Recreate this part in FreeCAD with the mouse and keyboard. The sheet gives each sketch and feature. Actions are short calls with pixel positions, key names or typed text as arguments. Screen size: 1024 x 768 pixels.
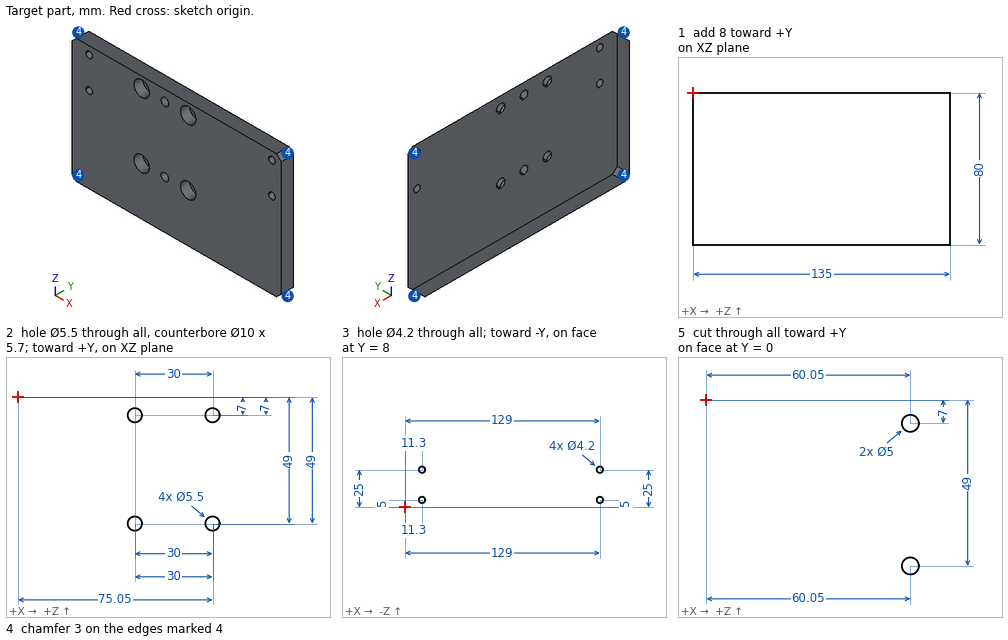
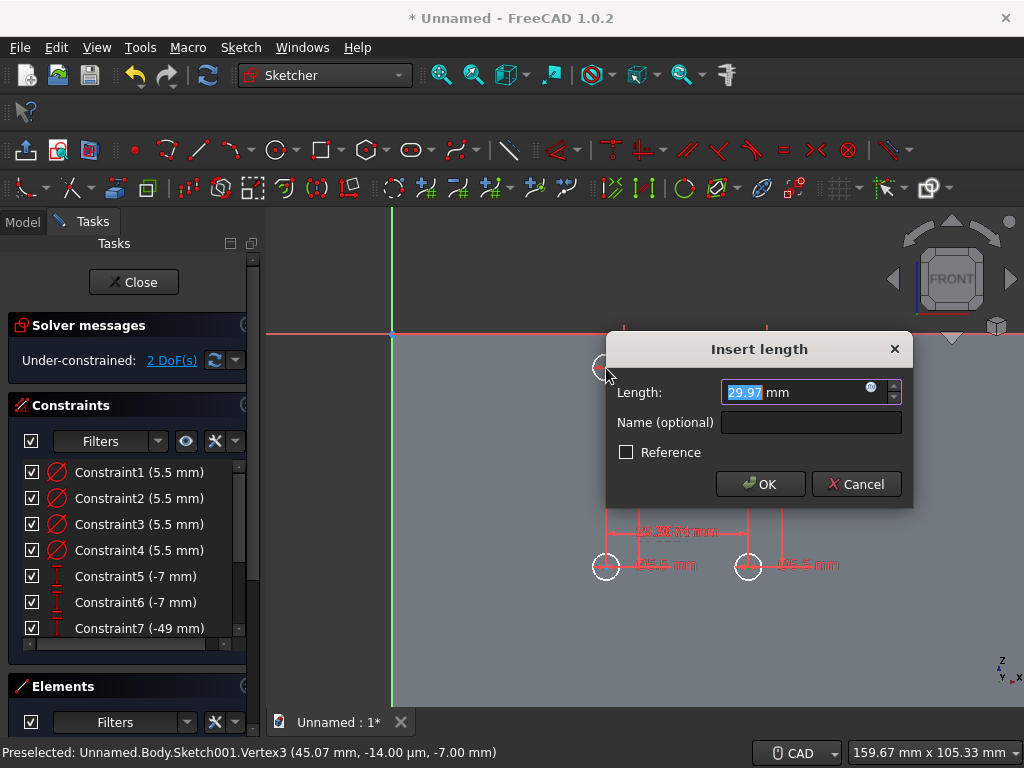
text(30)
key(Return)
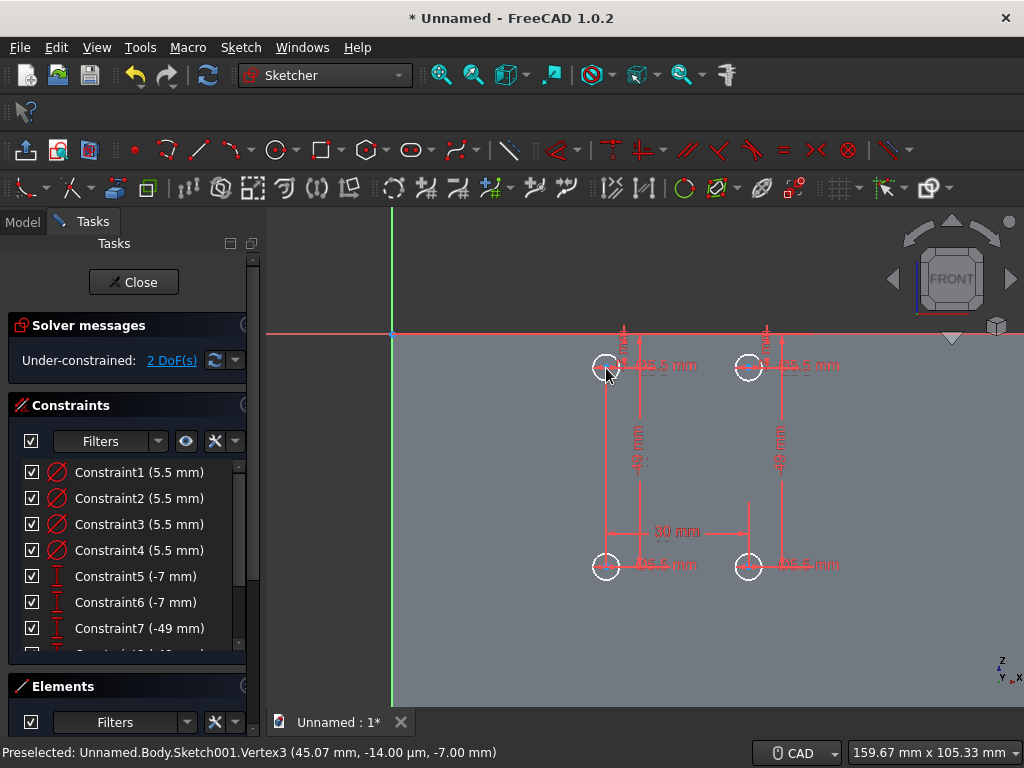
click(606, 368)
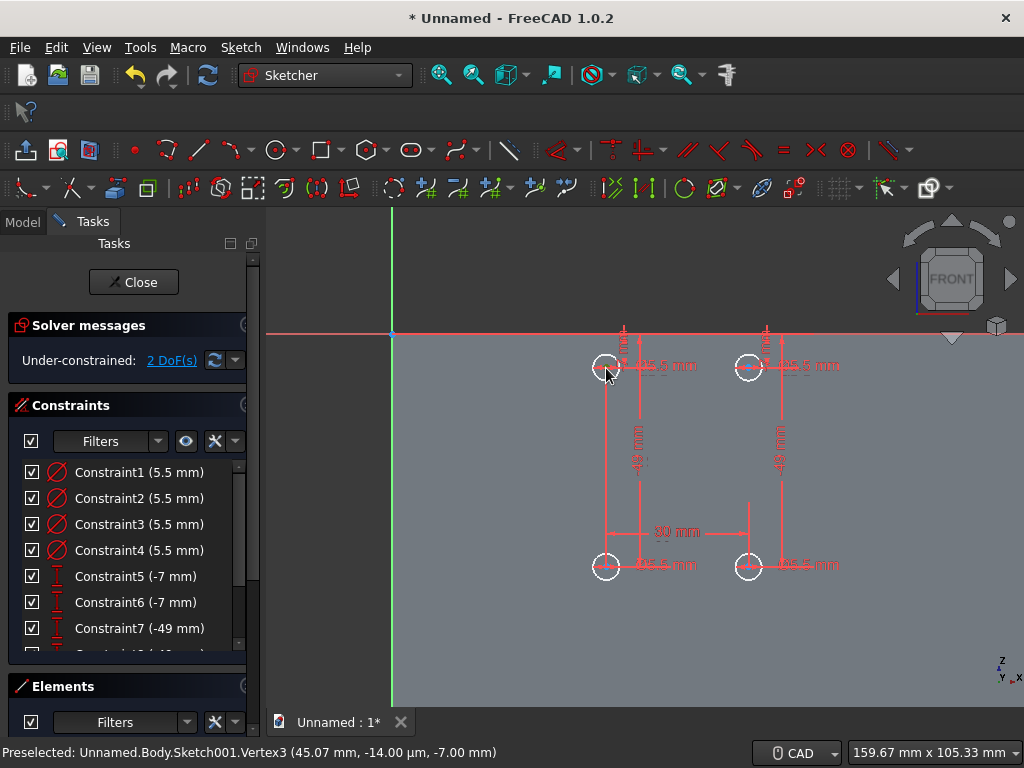
click(749, 368)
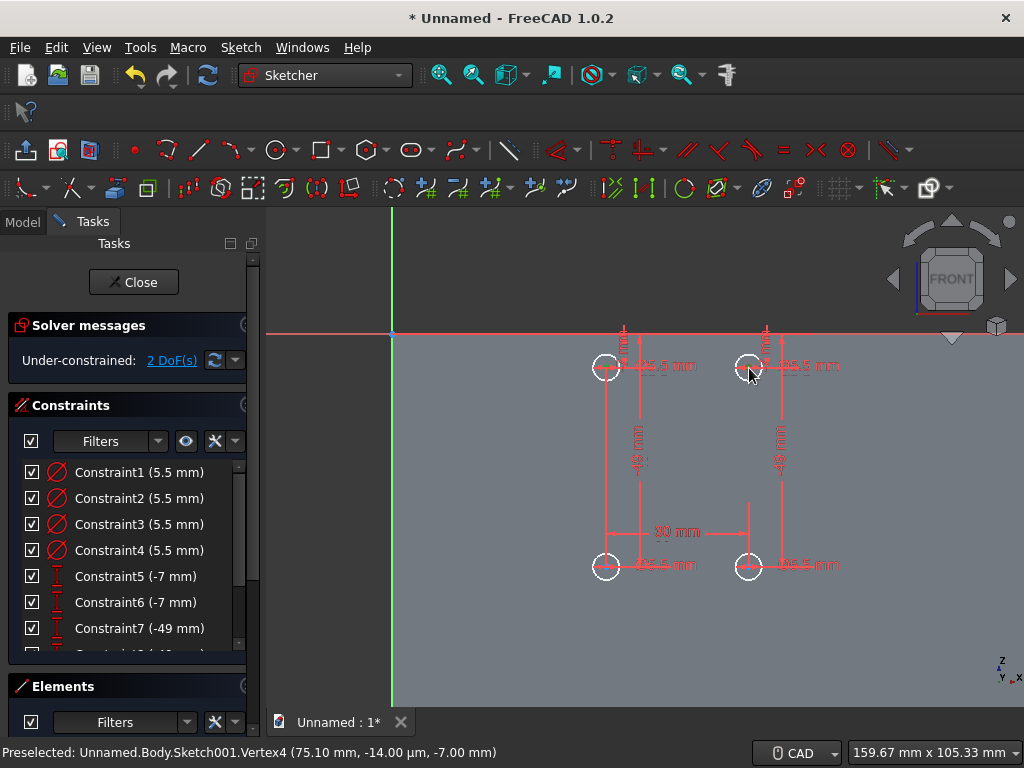
key(l)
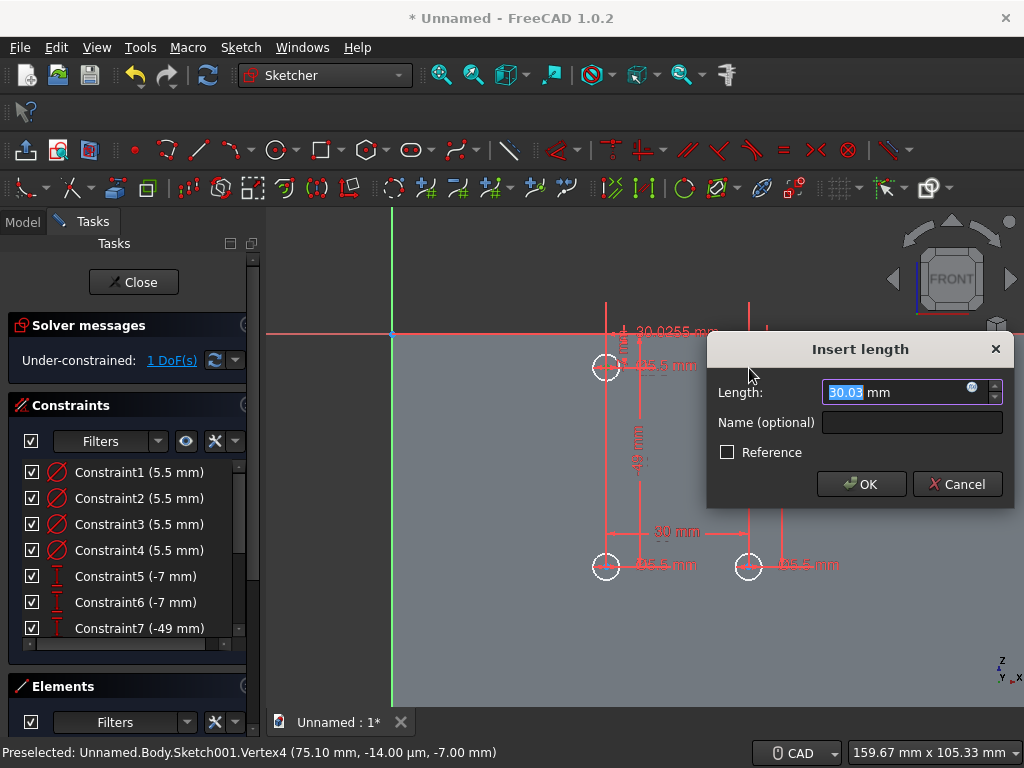
text(30)
key(Return)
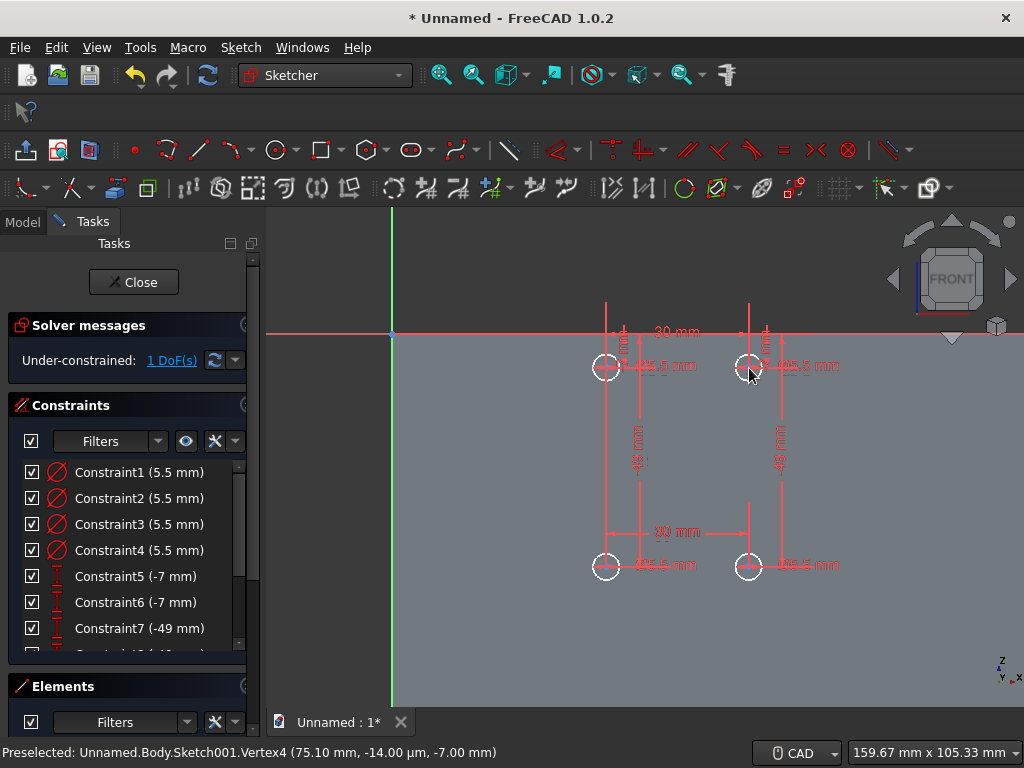
click(749, 567)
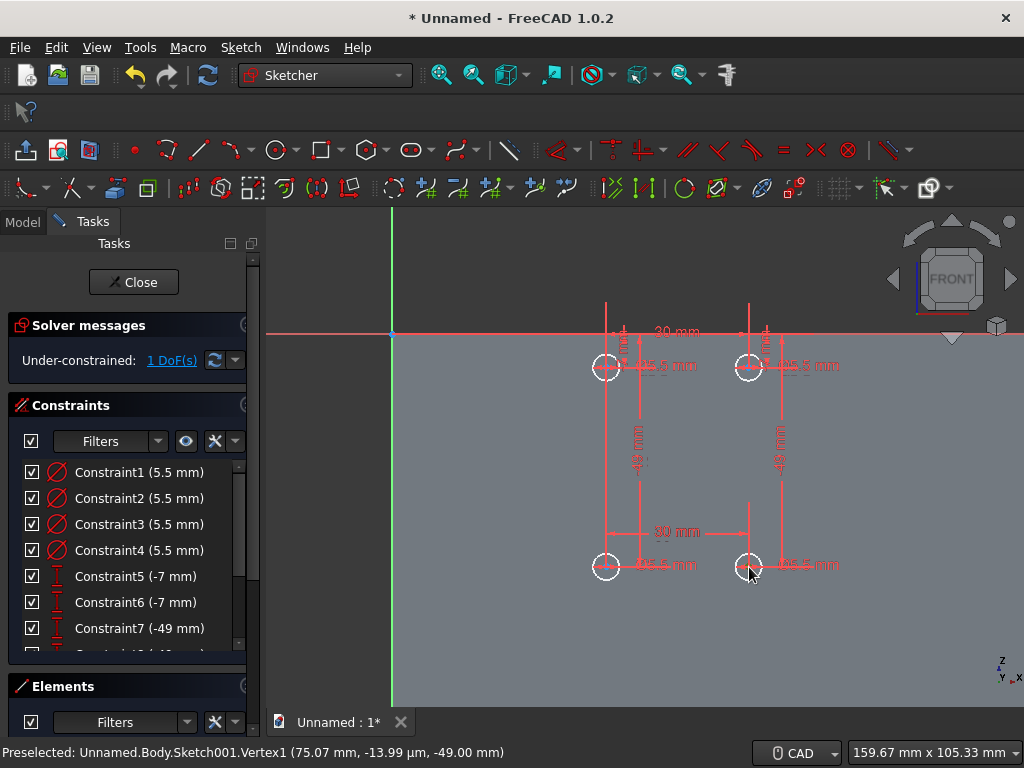
key(l)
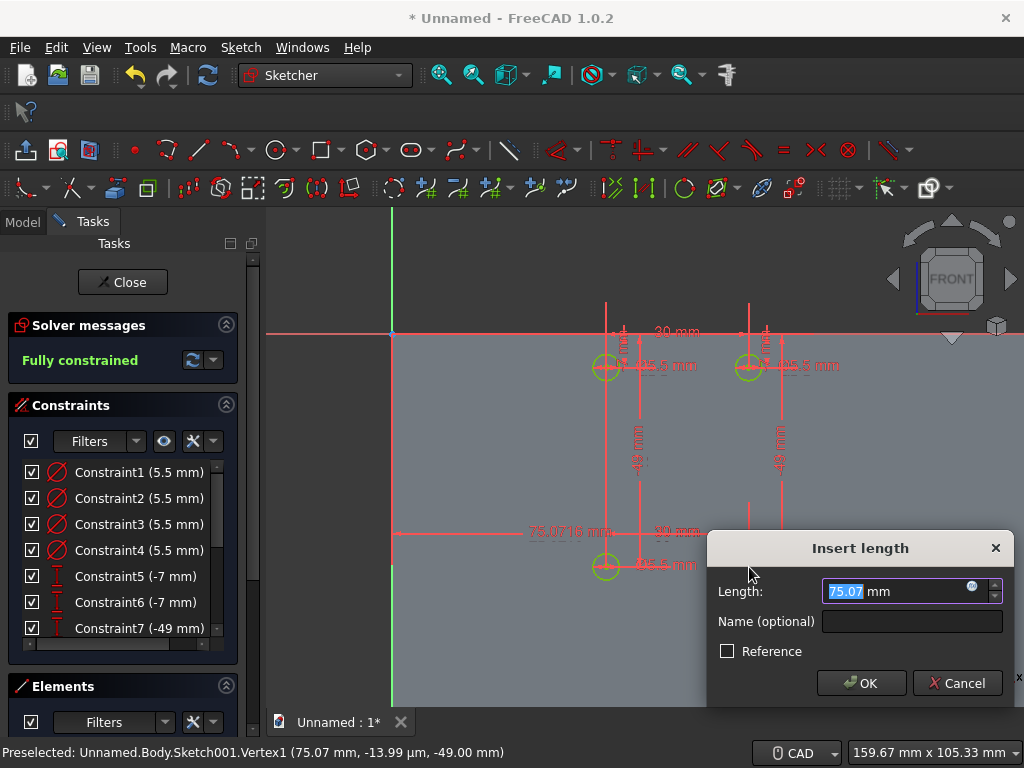
text(75.05)
key(Return)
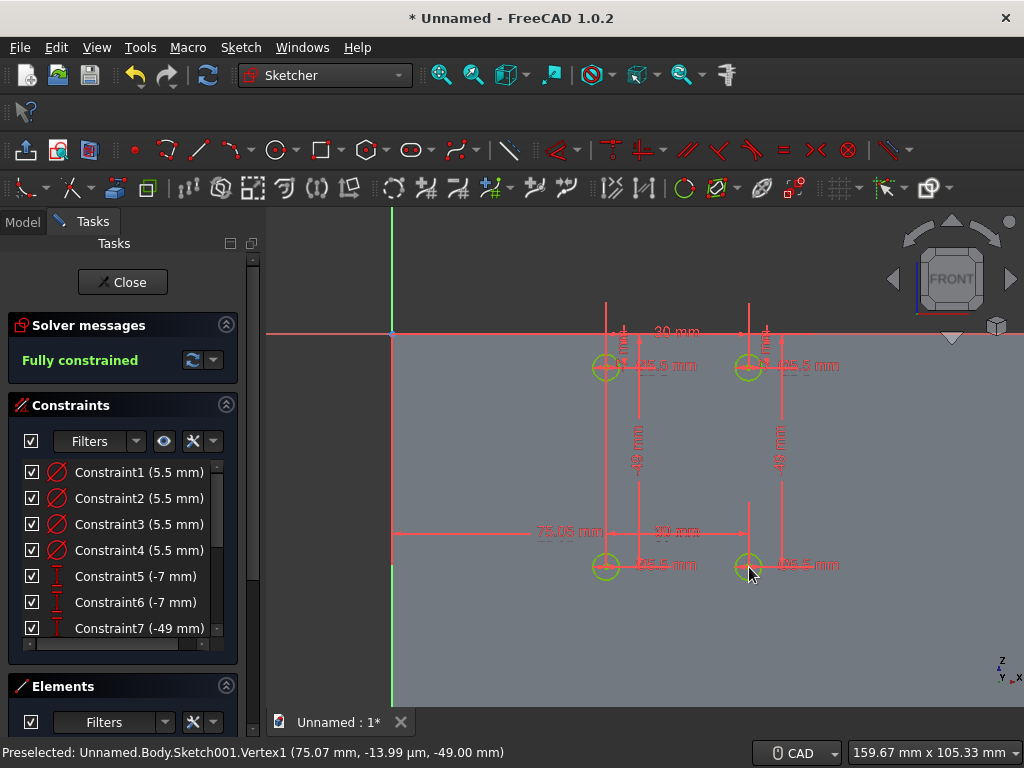
click(123, 282)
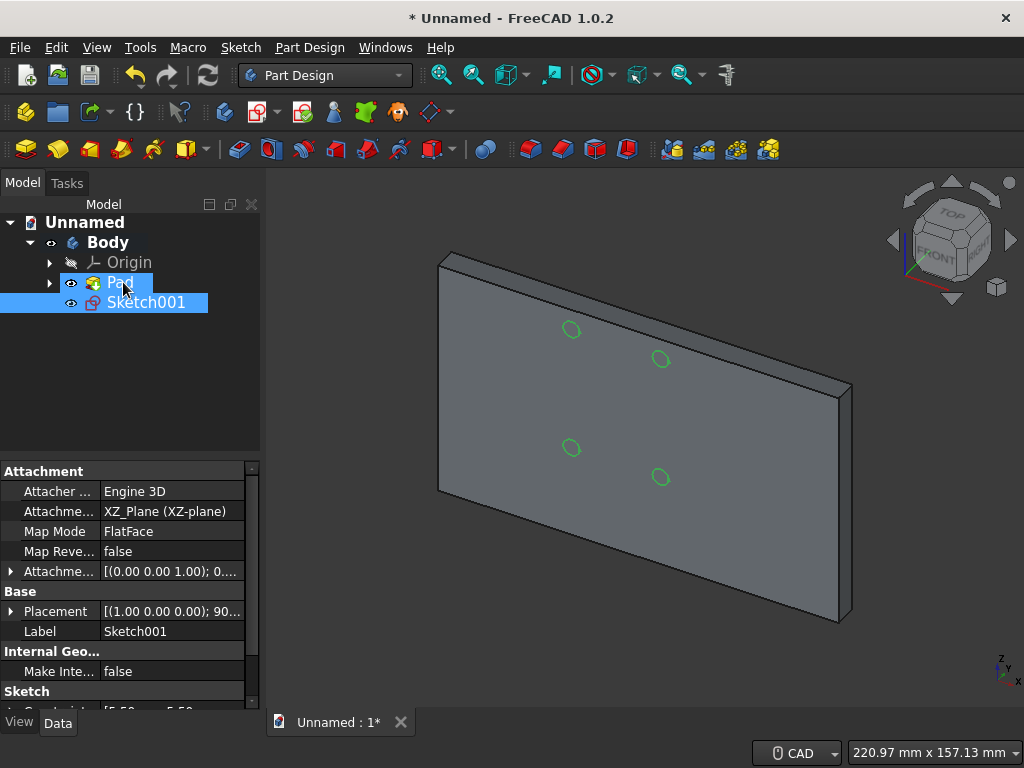
click(272, 150)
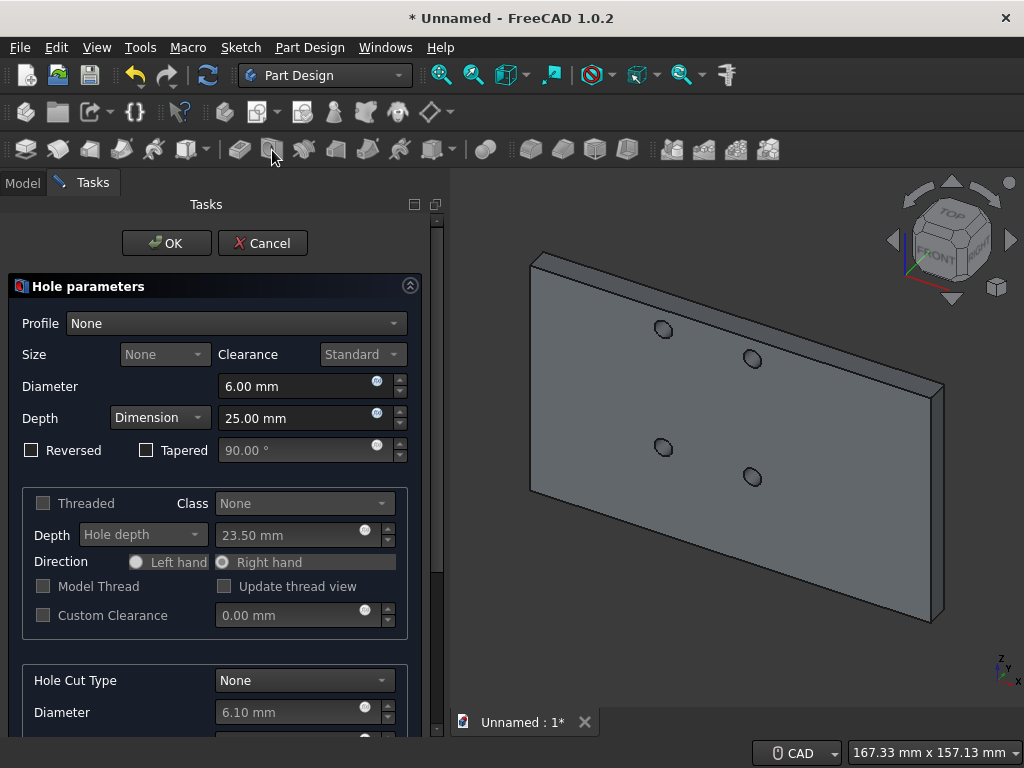
triple_click(305, 386)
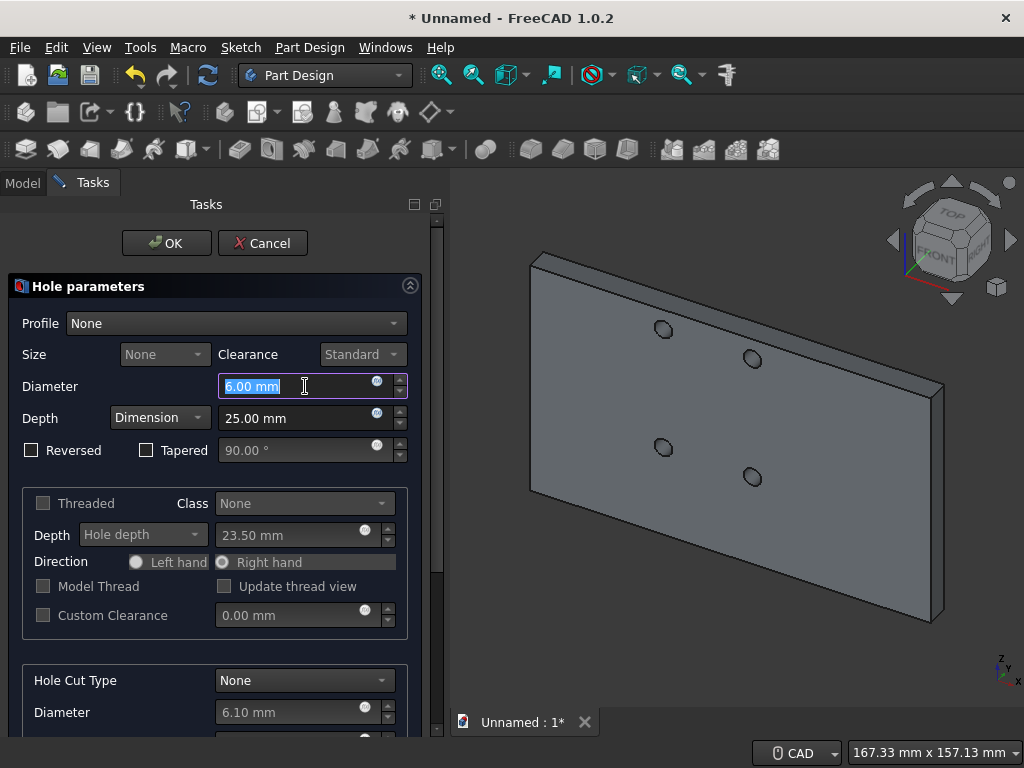
text(5.5)
key(Tab)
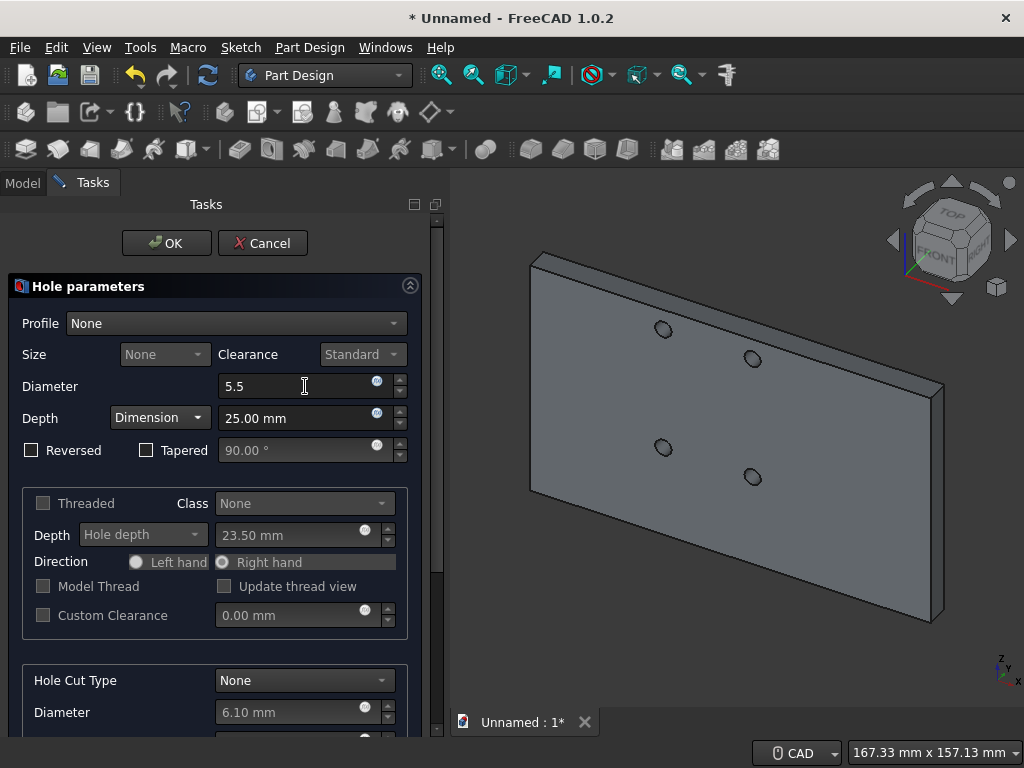
click(161, 418)